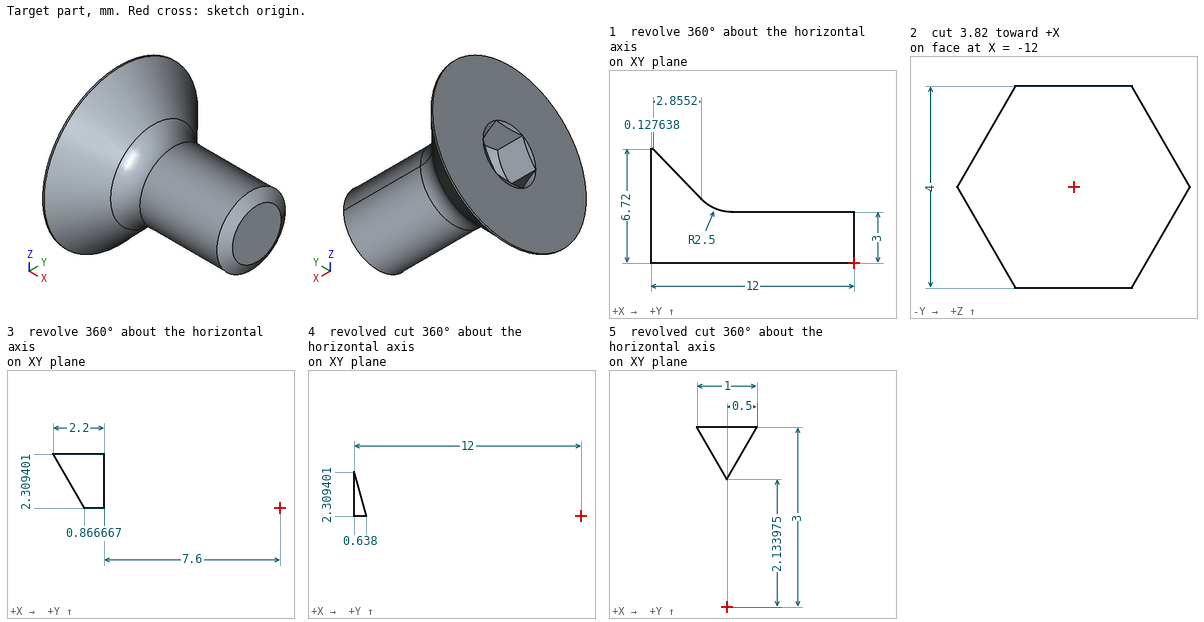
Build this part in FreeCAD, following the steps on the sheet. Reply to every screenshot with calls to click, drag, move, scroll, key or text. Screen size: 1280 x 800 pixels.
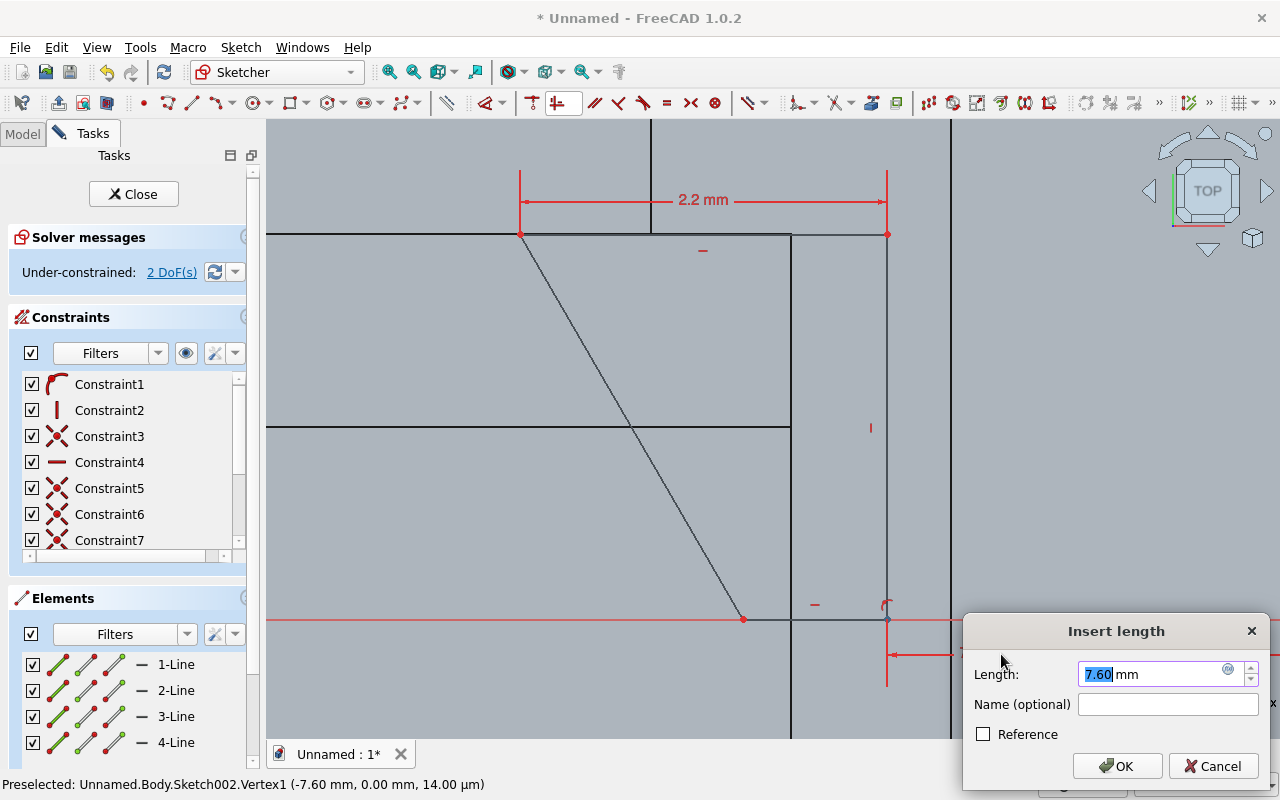
text(7.6)
key(Return)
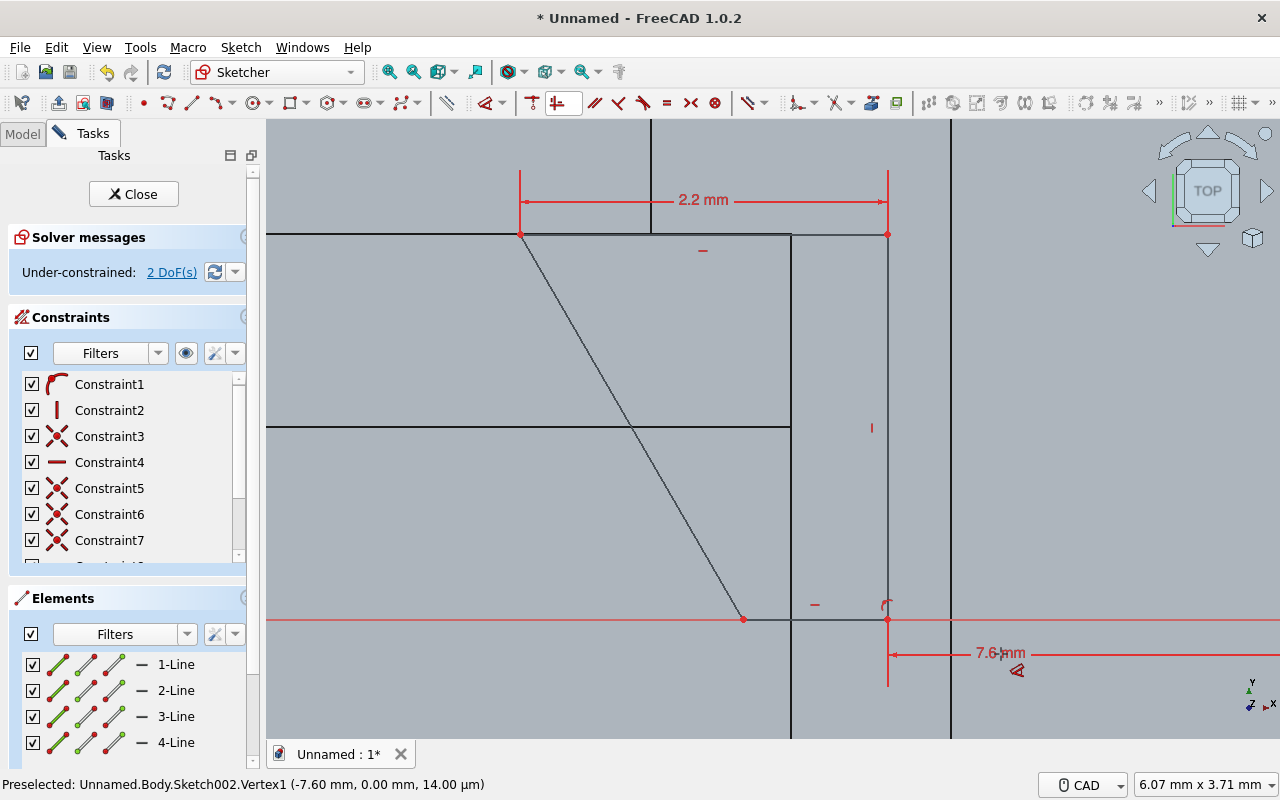
click(888, 504)
click(922, 427)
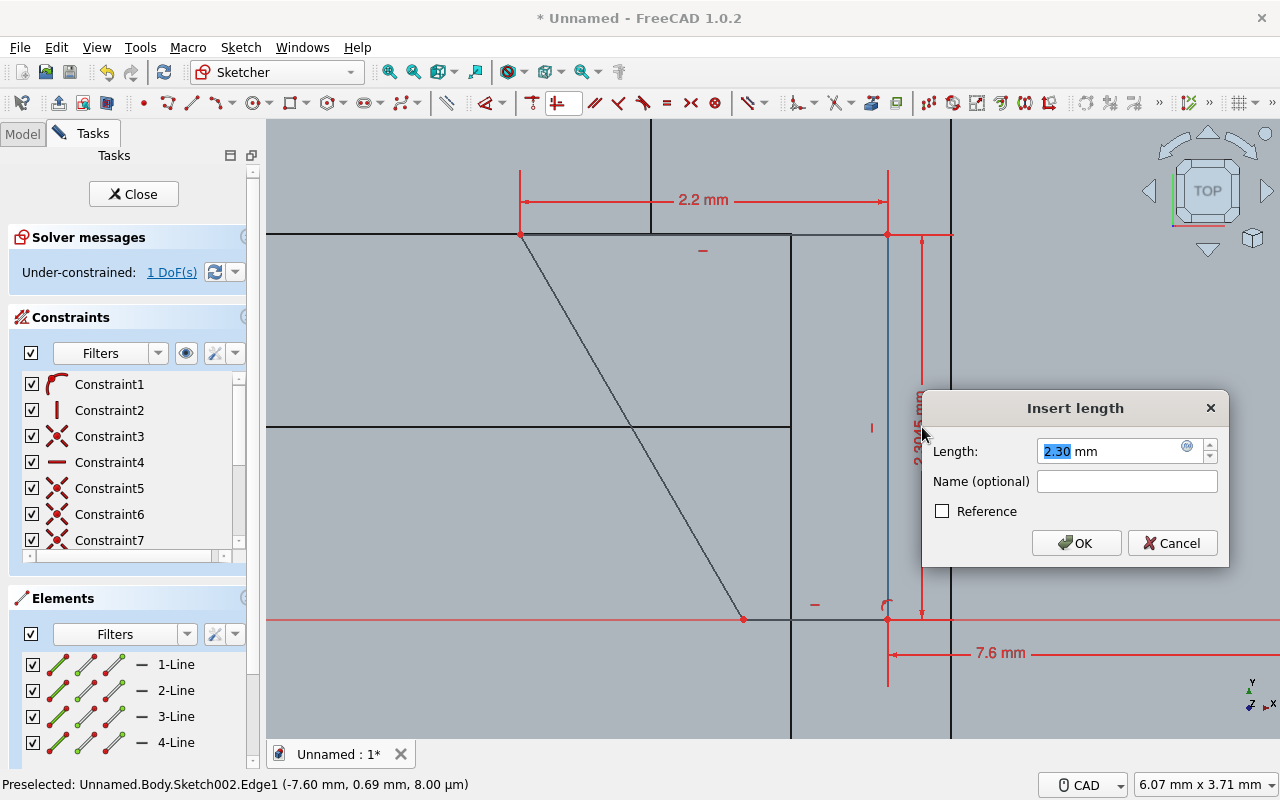
text(2.309401)
key(Return)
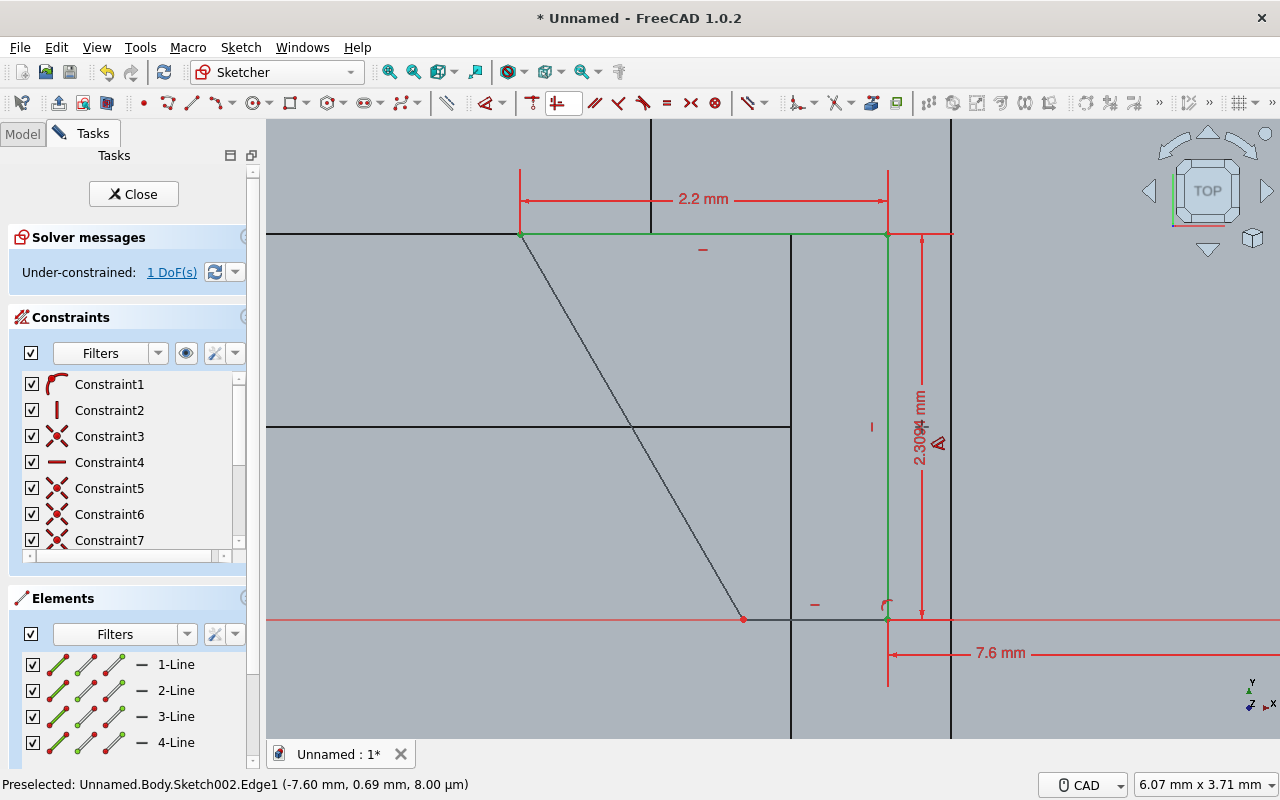
click(786, 620)
click(815, 654)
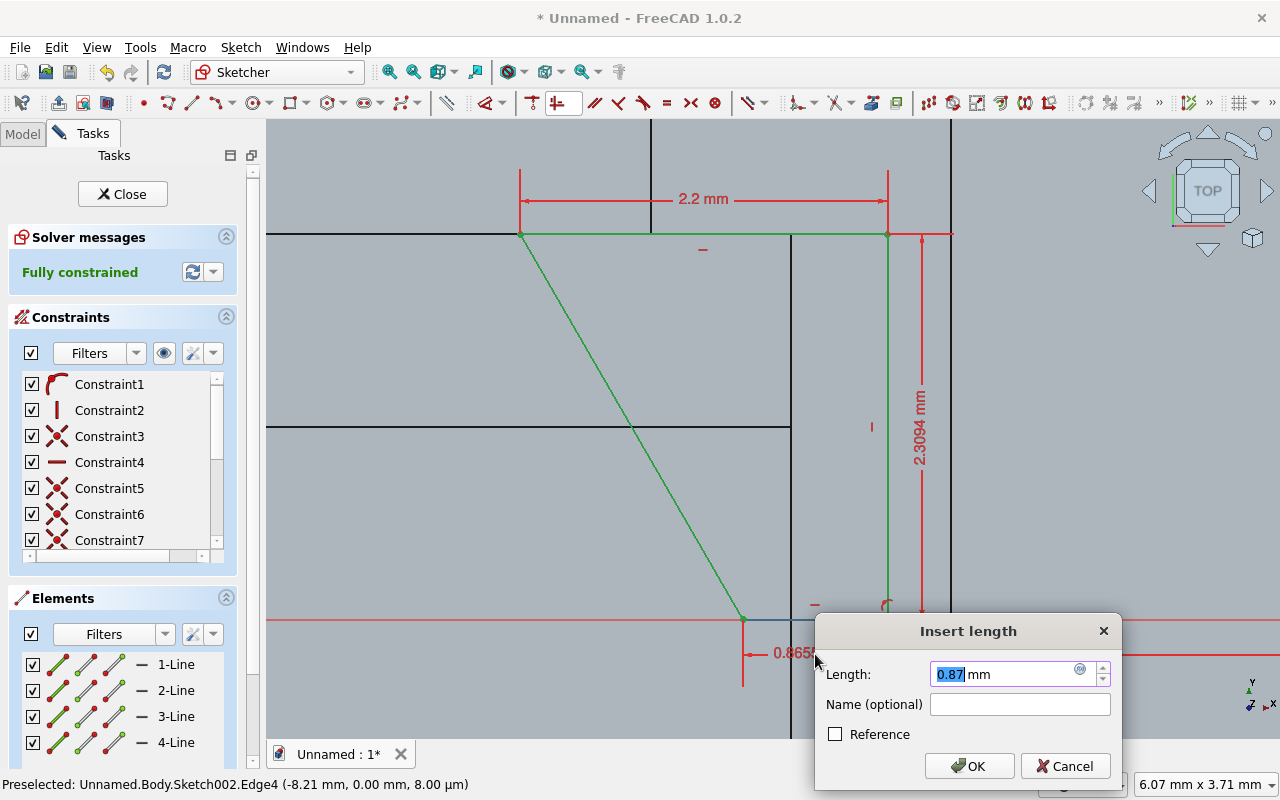
text(0.866667)
key(Return)
key(Escape)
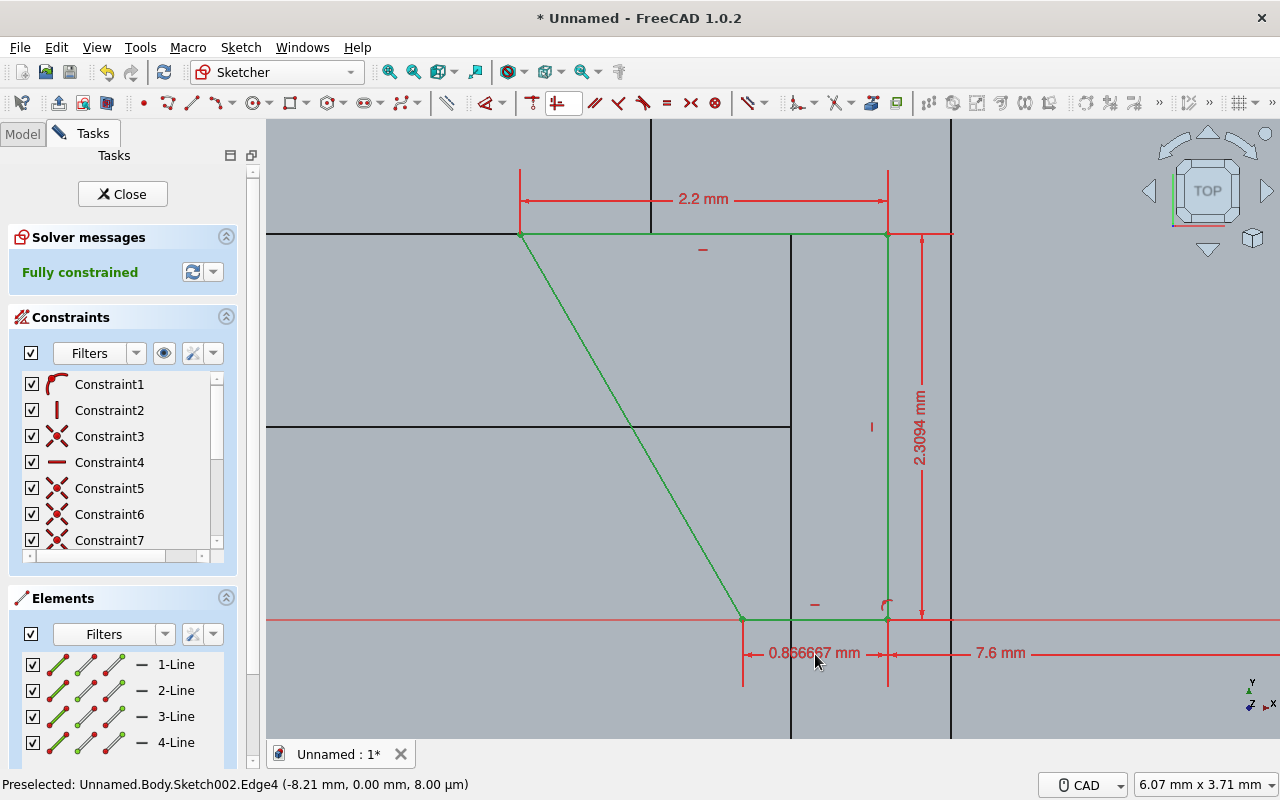
click(123, 194)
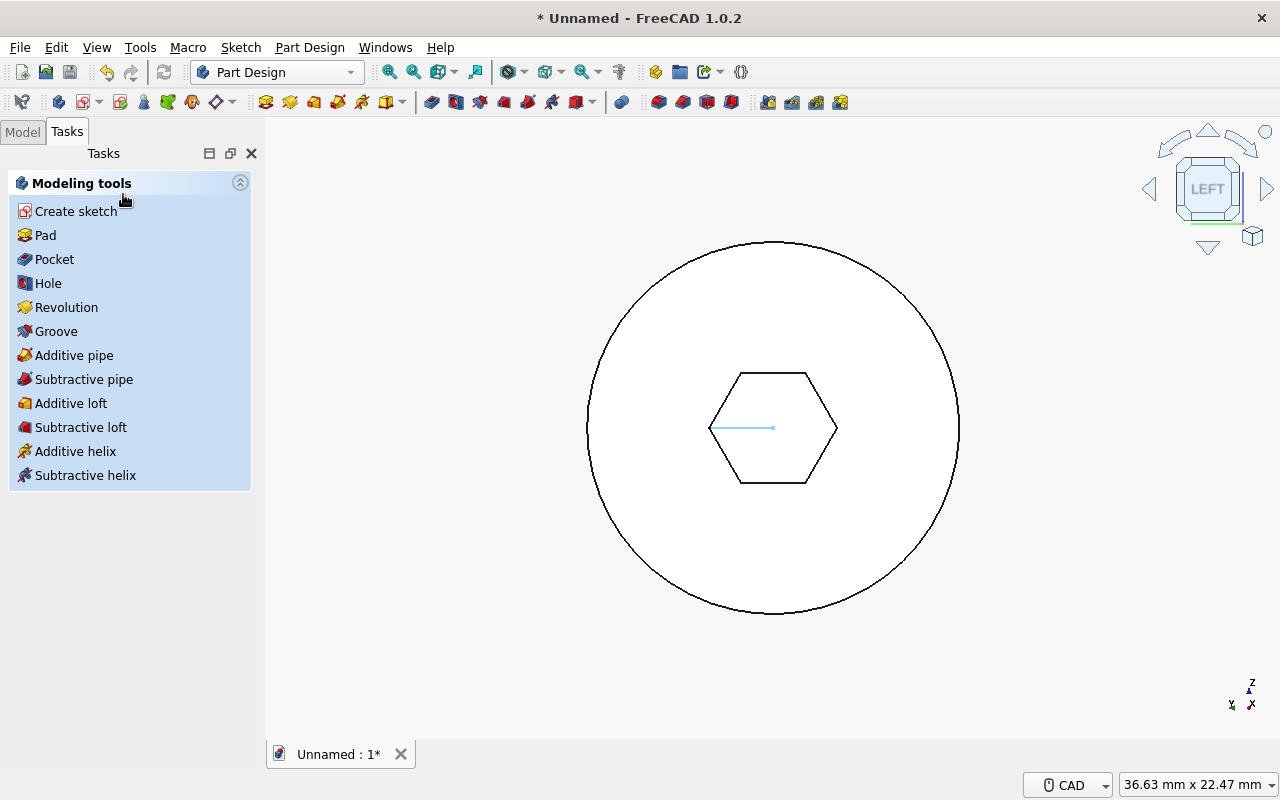
click(290, 102)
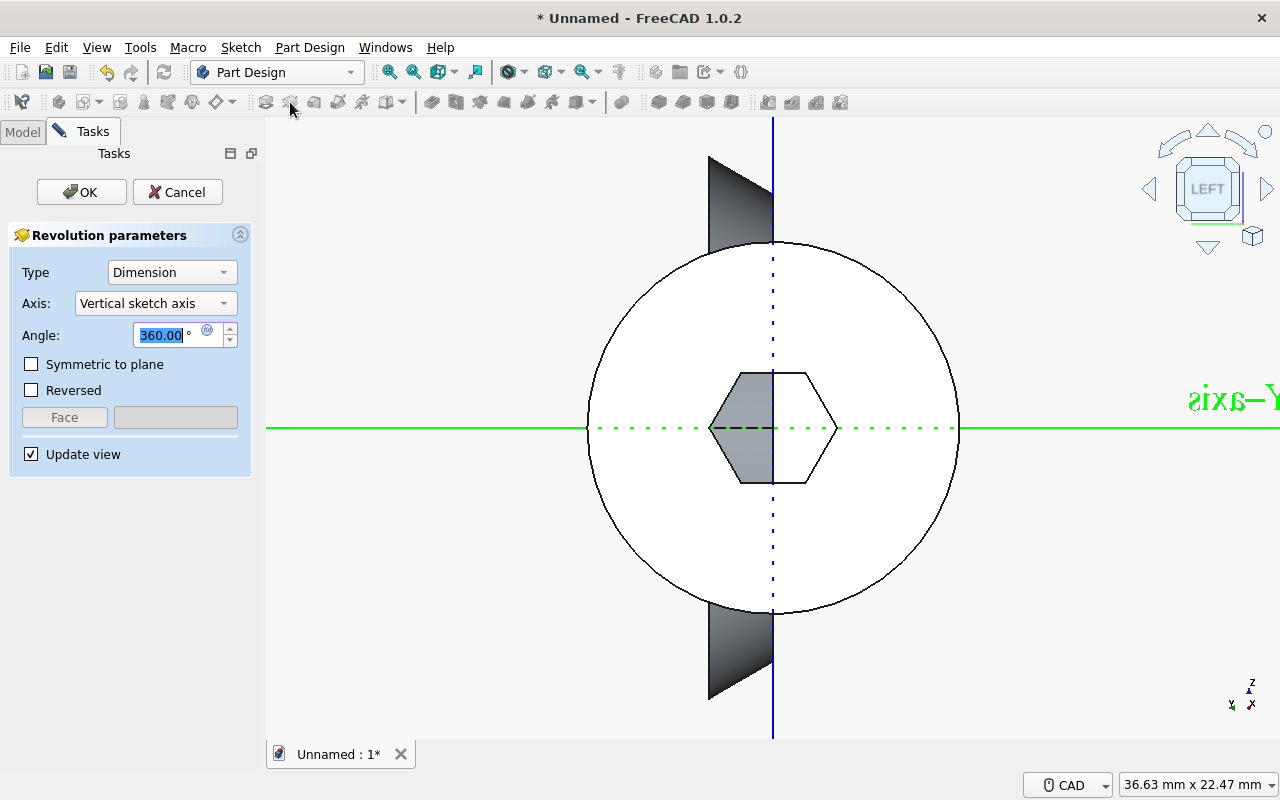
click(156, 304)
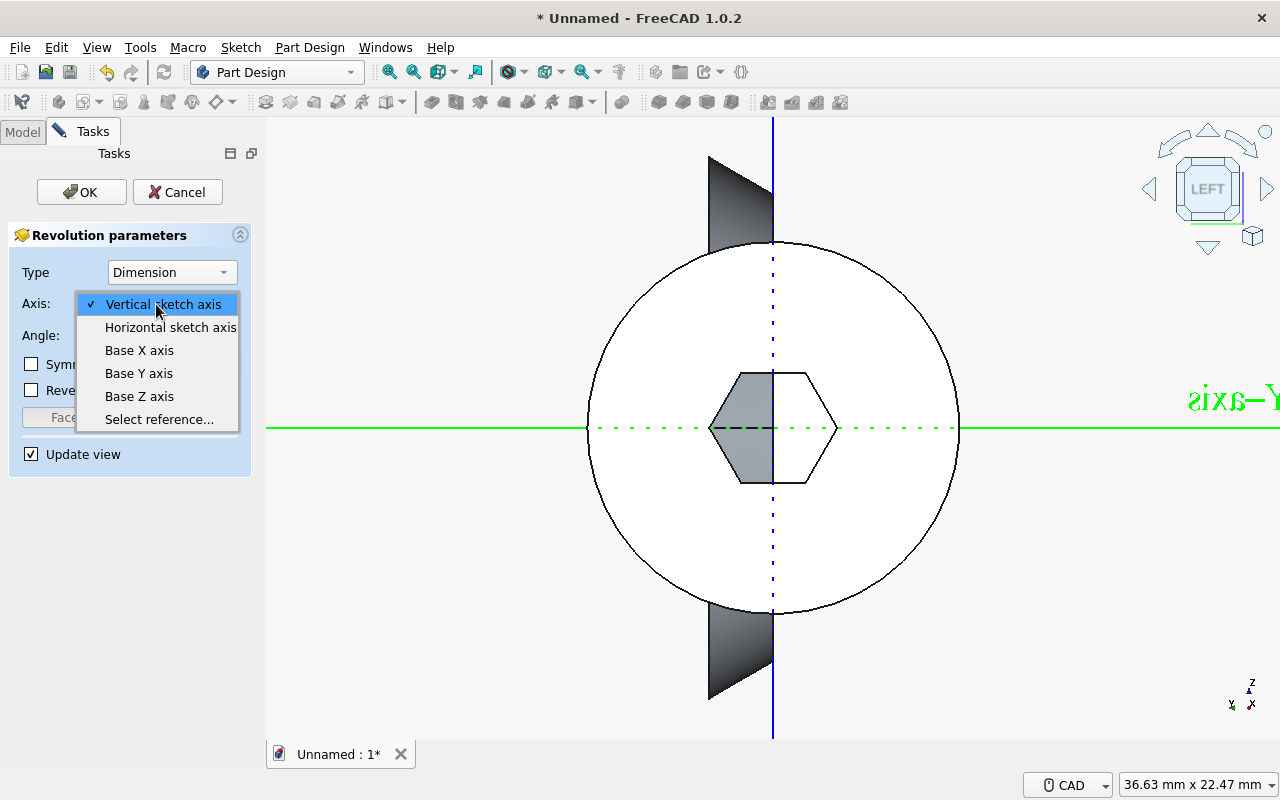
click(156, 328)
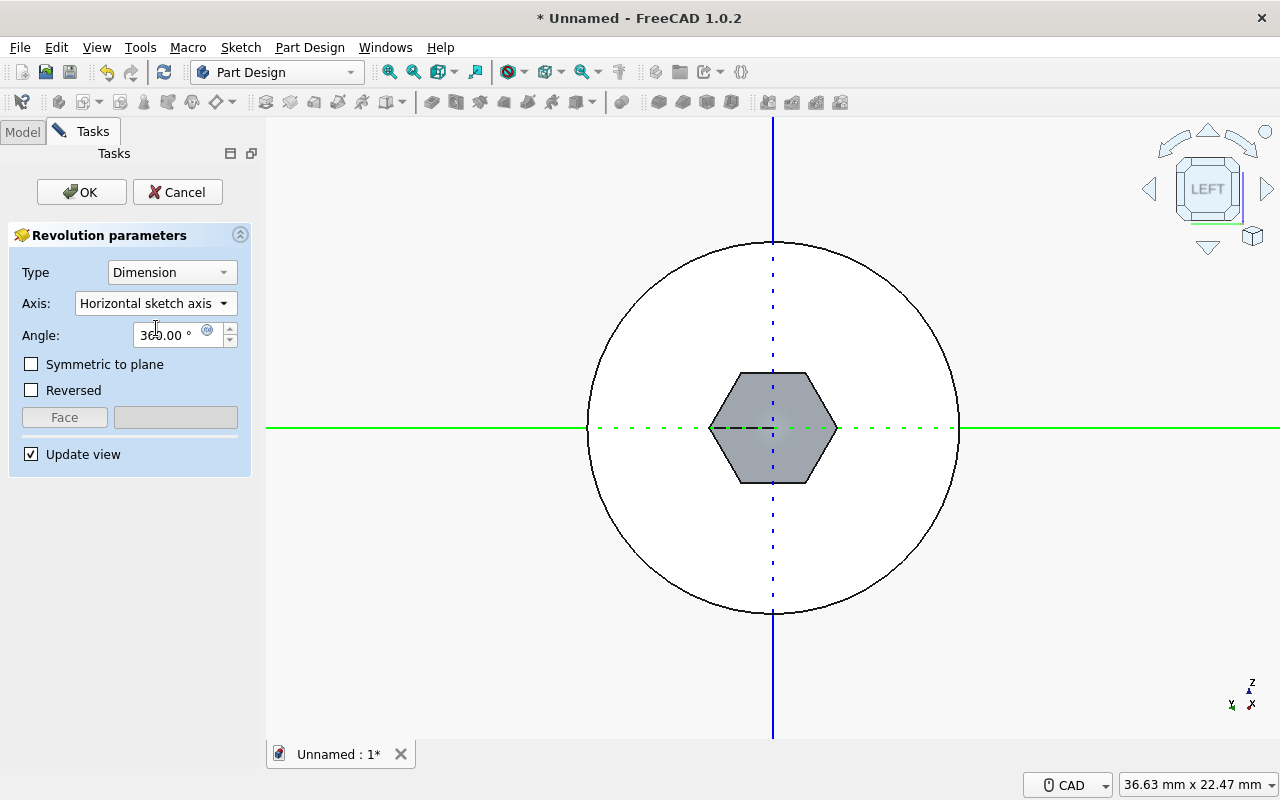
click(82, 192)